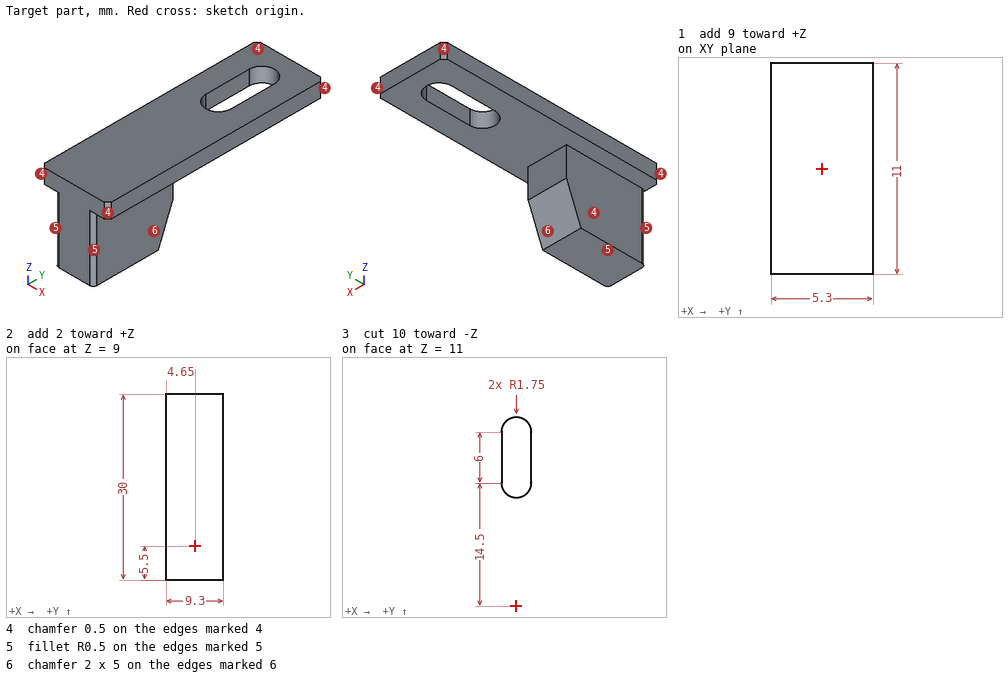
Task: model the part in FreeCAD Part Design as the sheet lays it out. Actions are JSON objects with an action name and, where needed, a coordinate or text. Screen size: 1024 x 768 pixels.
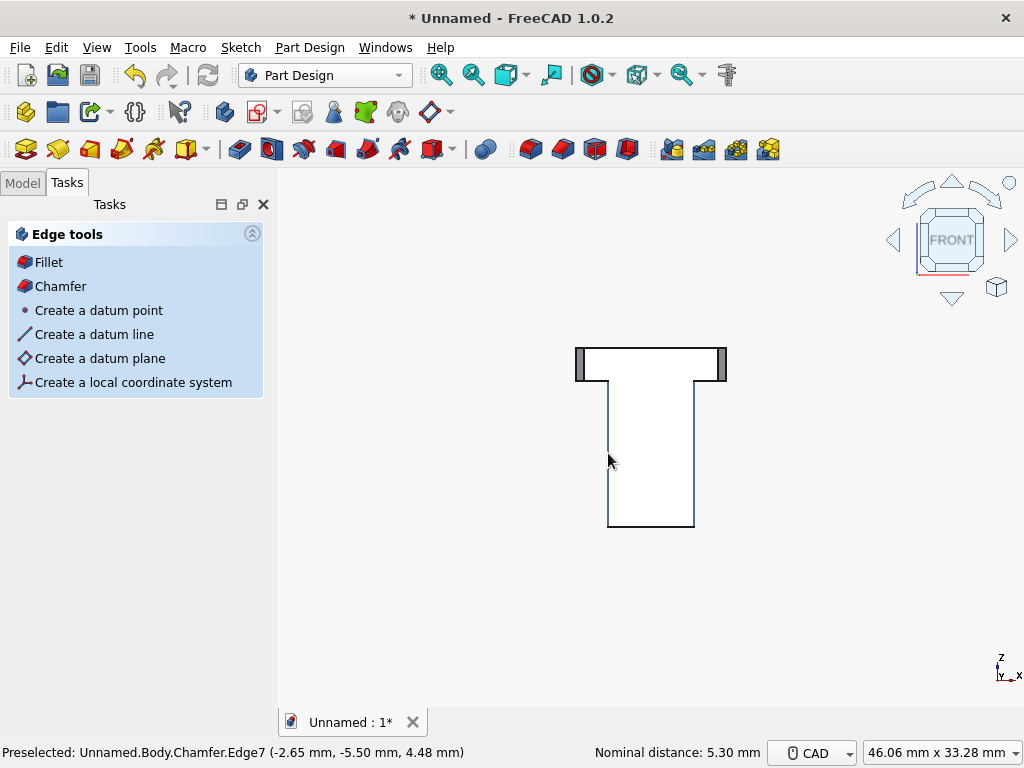
{"action": "left_click", "coordinate": [532, 150]}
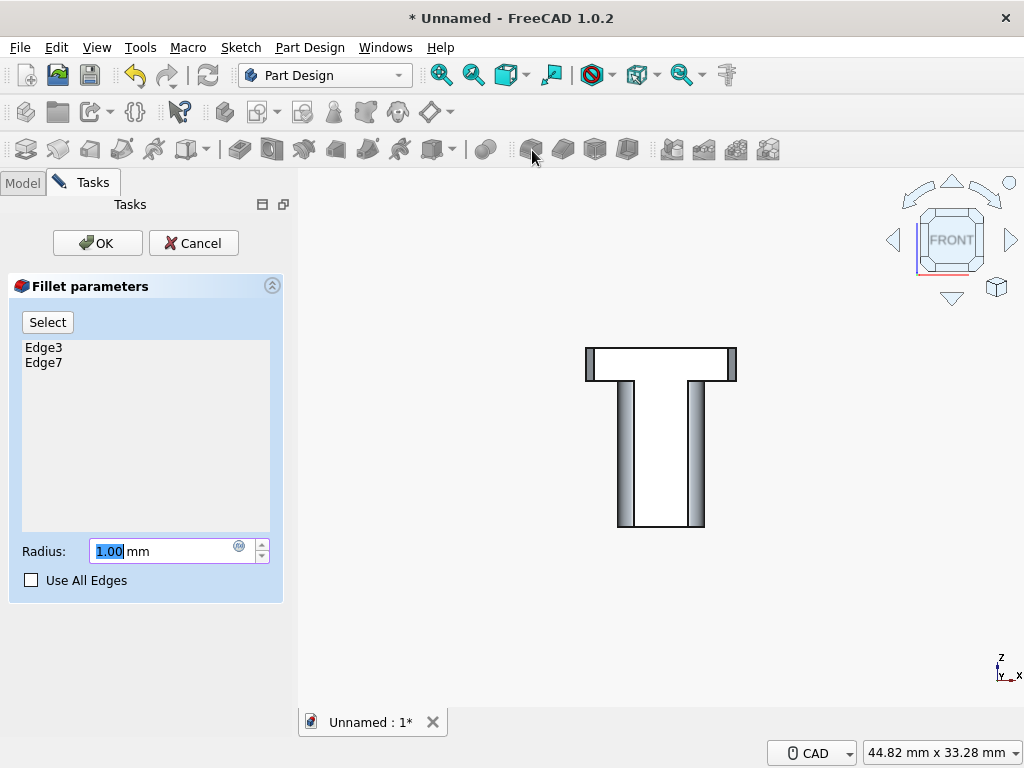
{"action": "type", "text": "0.5"}
{"action": "key", "text": "Tab"}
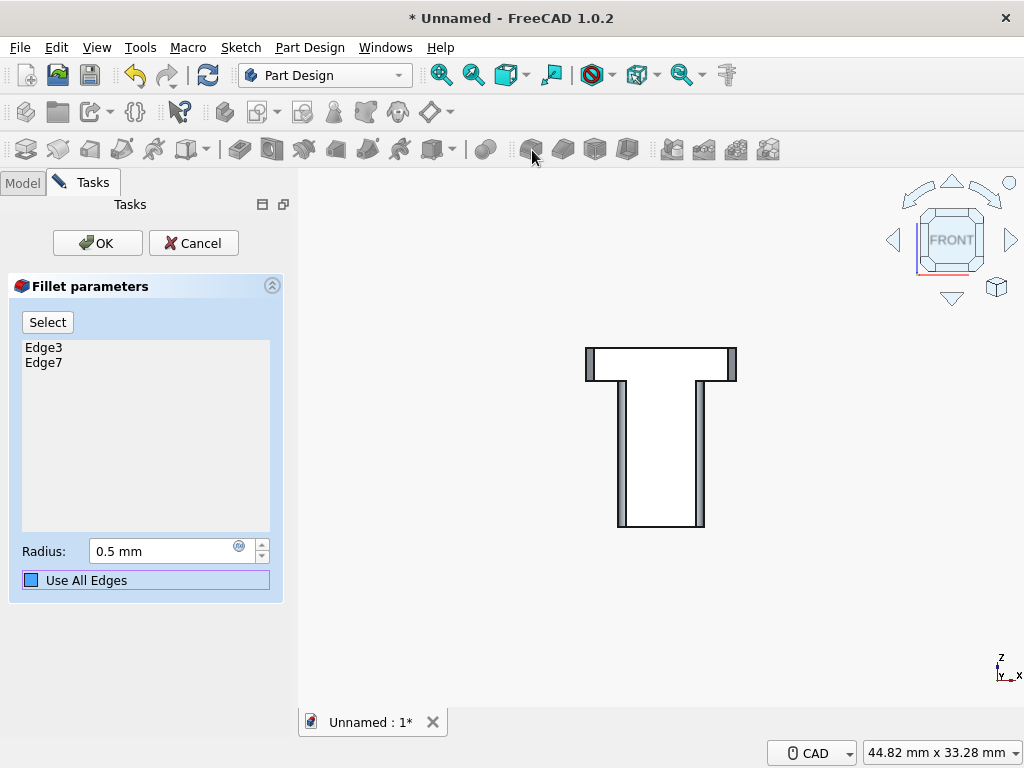
{"action": "left_click", "coordinate": [98, 243]}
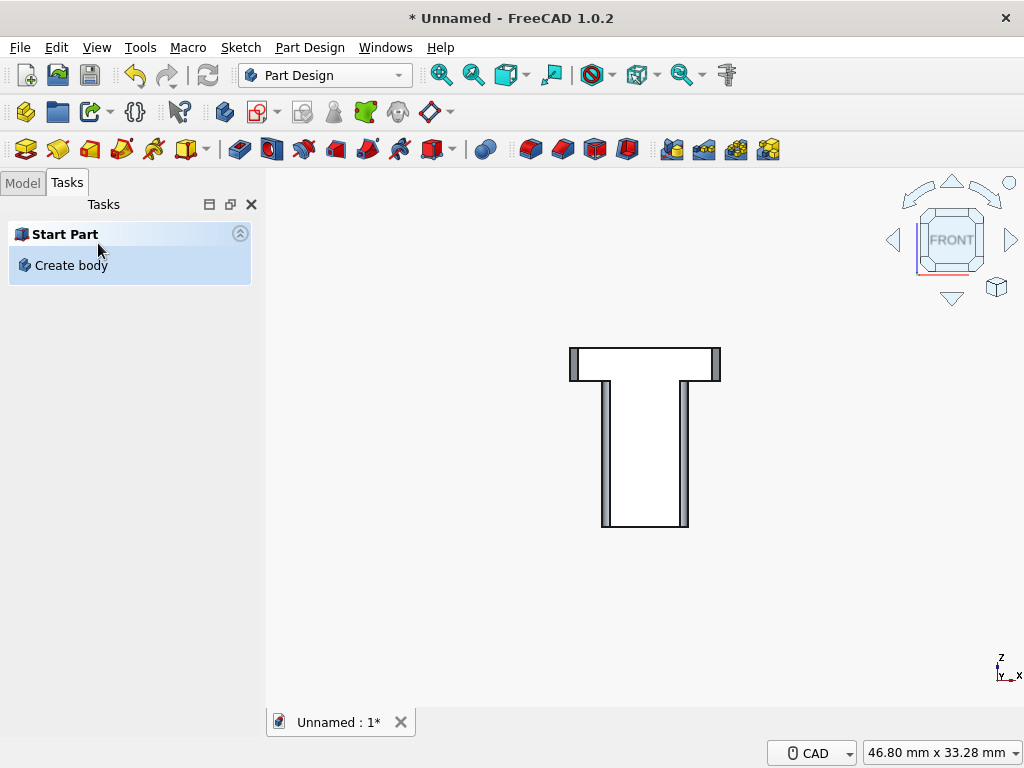
{"action": "key", "text": "v f"}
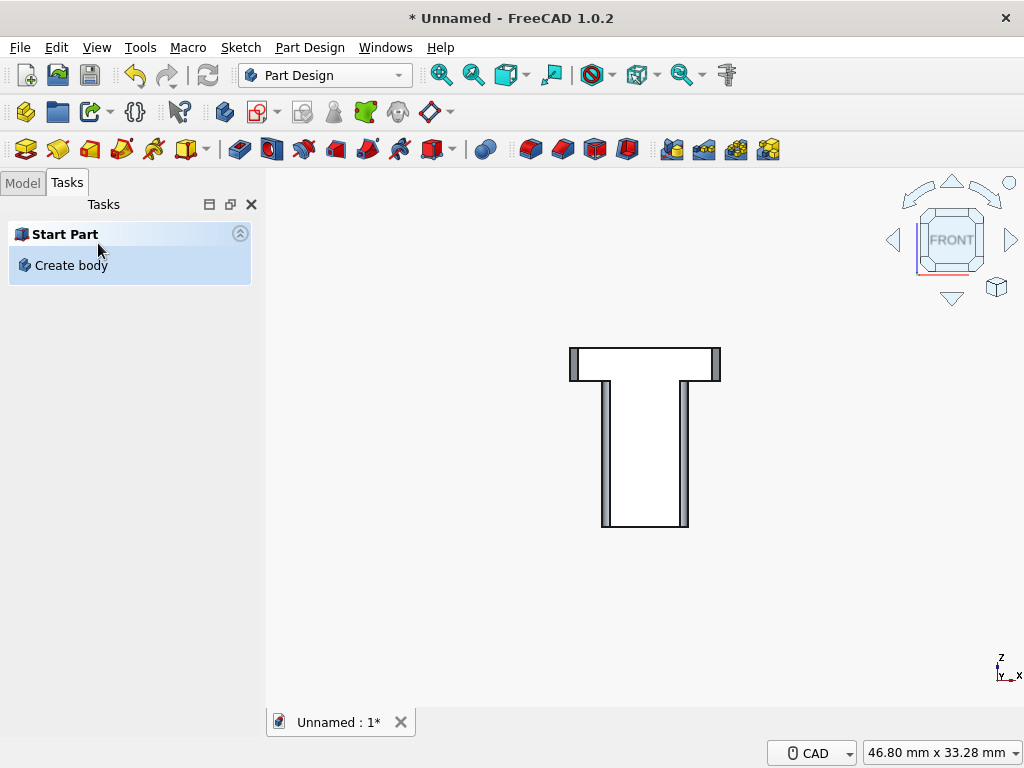
{"action": "key", "text": "0"}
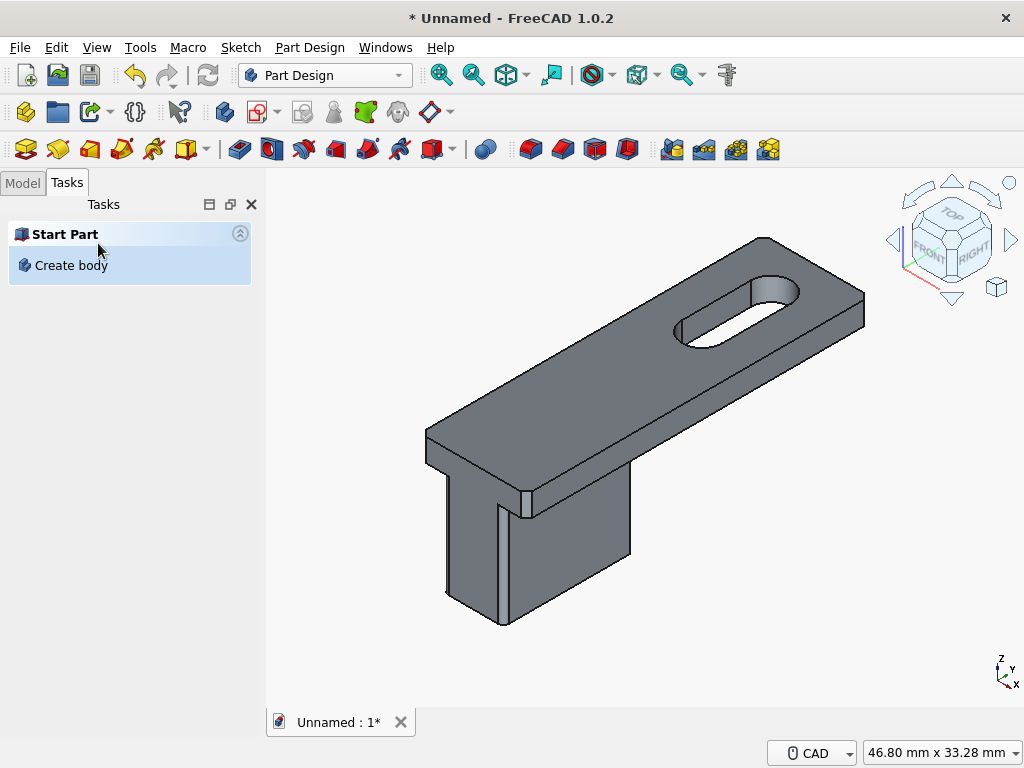
{"action": "key", "text": "2"}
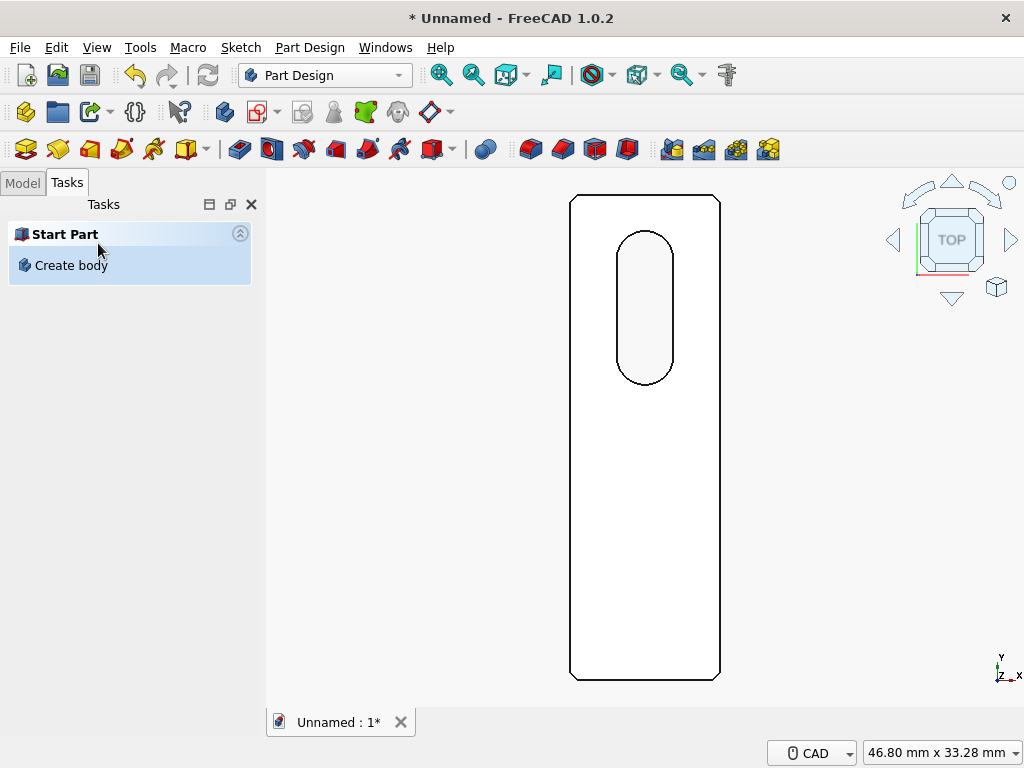
{"action": "key", "text": "1"}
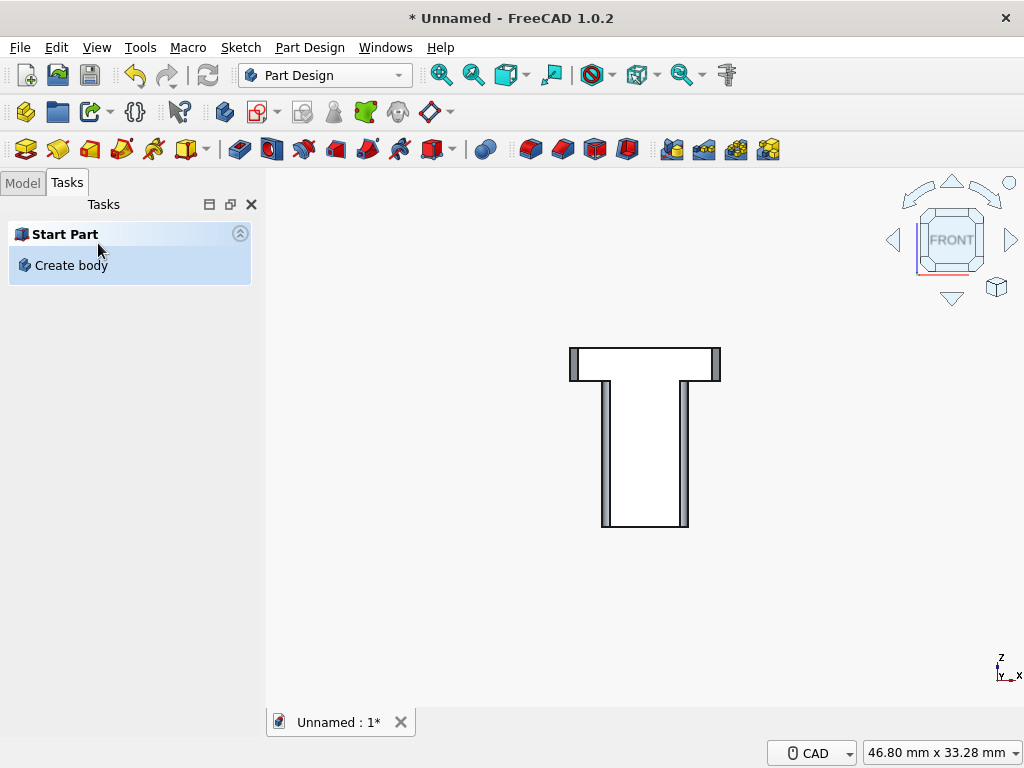
{"action": "left_click", "coordinate": [442, 76]}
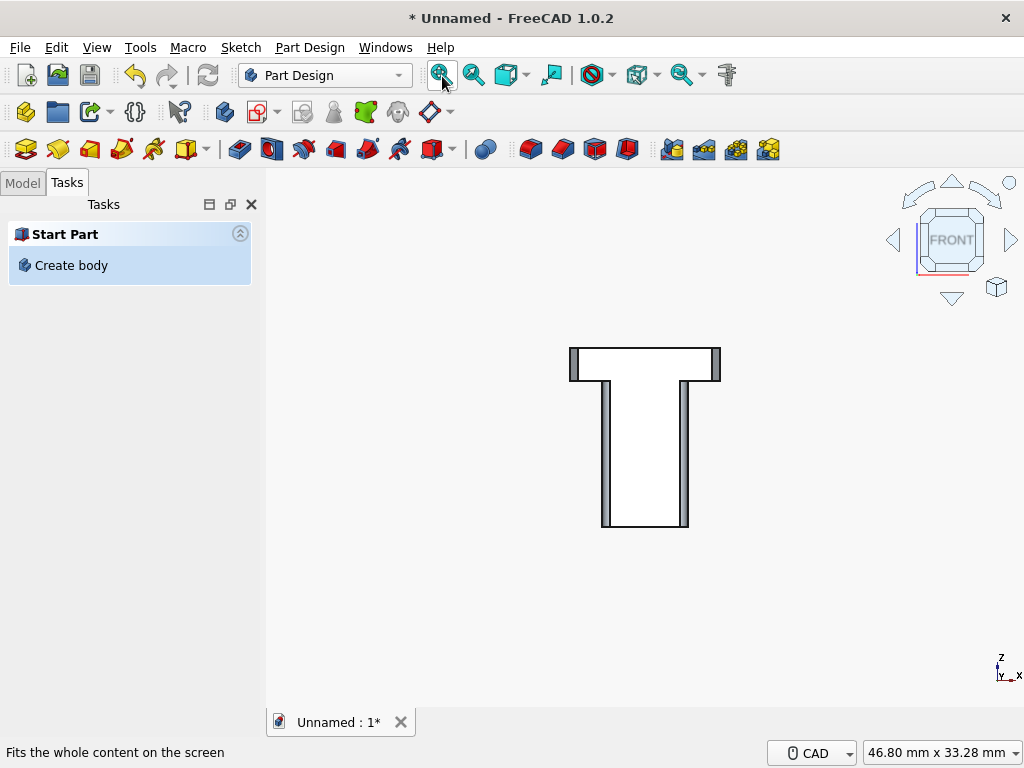
{"action": "key", "text": "3"}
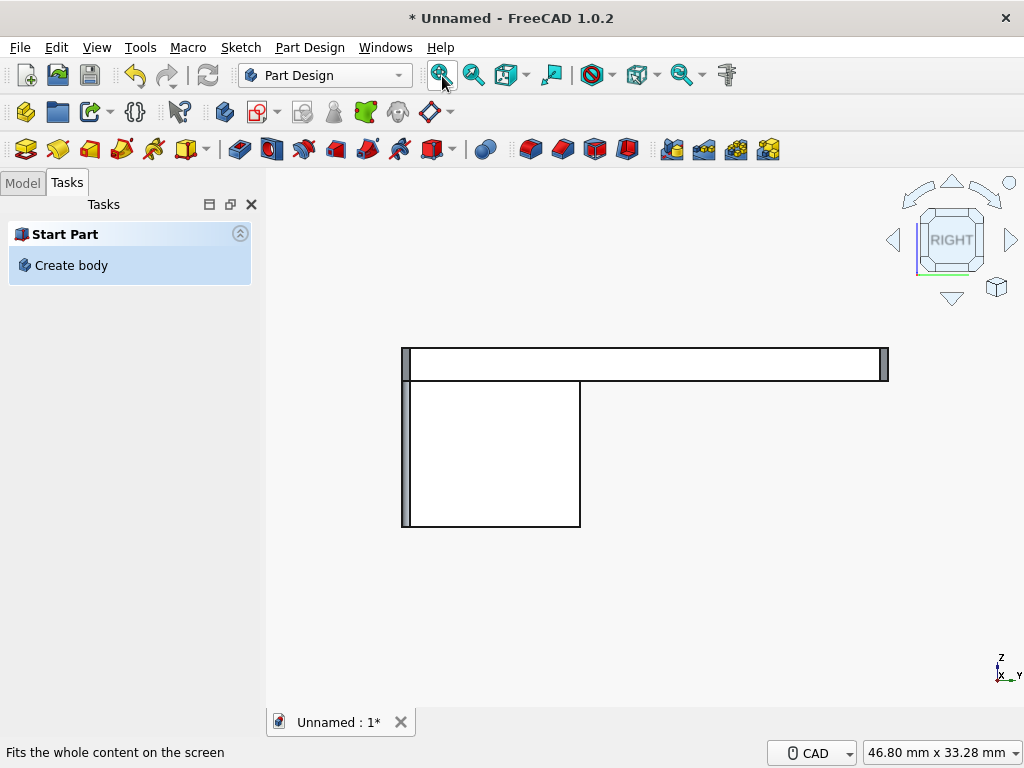
{"action": "key", "text": "5"}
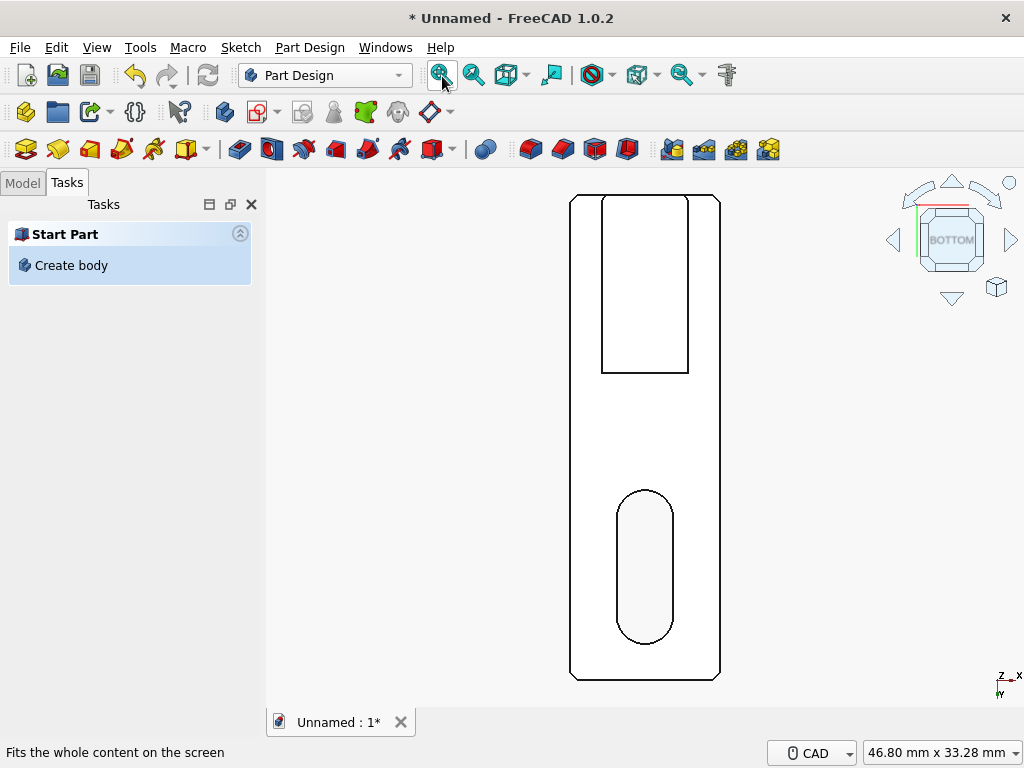
{"action": "left_click", "coordinate": [645, 372]}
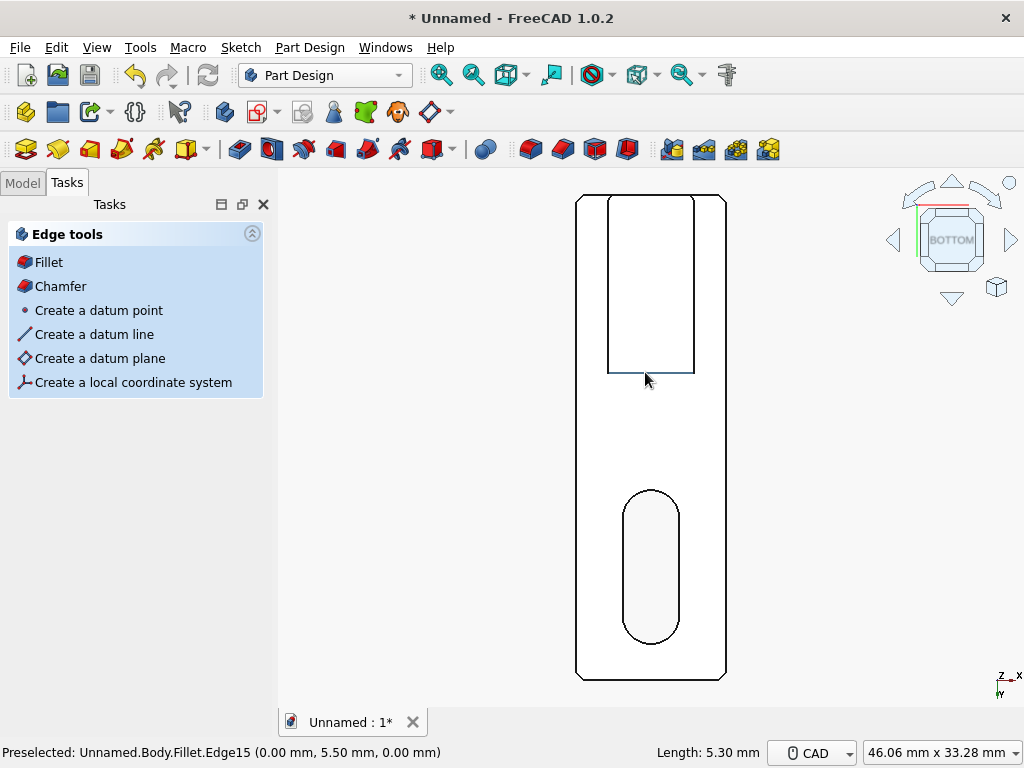
{"action": "left_click", "coordinate": [564, 150]}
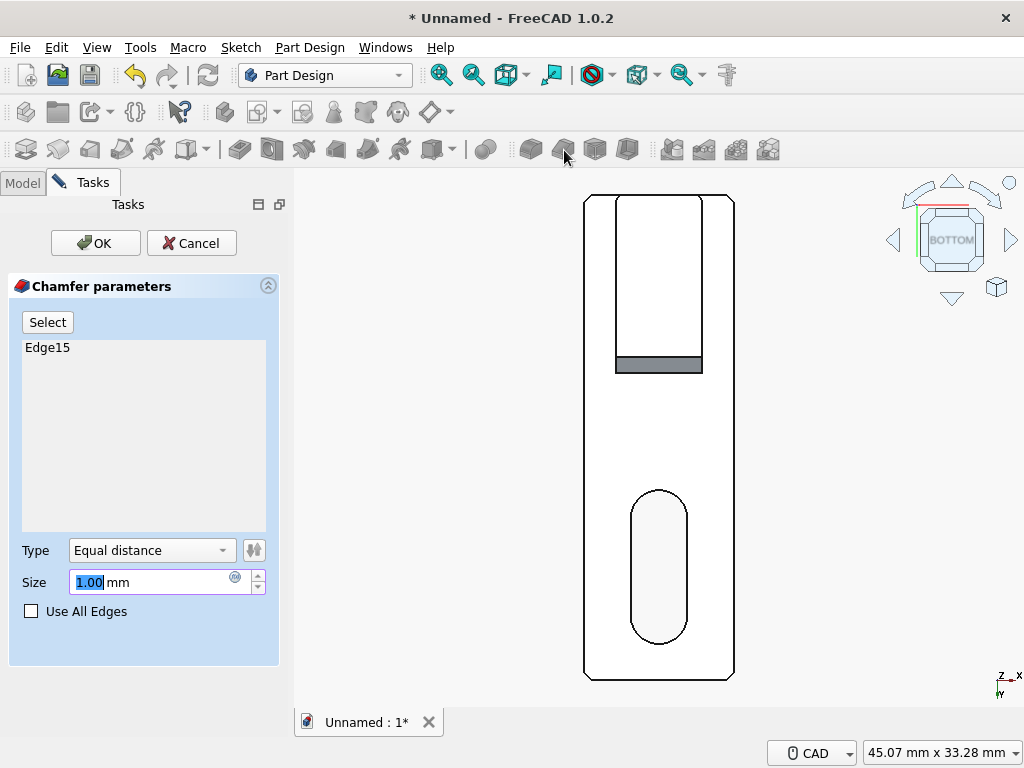
{"action": "type", "text": "2"}
{"action": "key", "text": "Tab"}